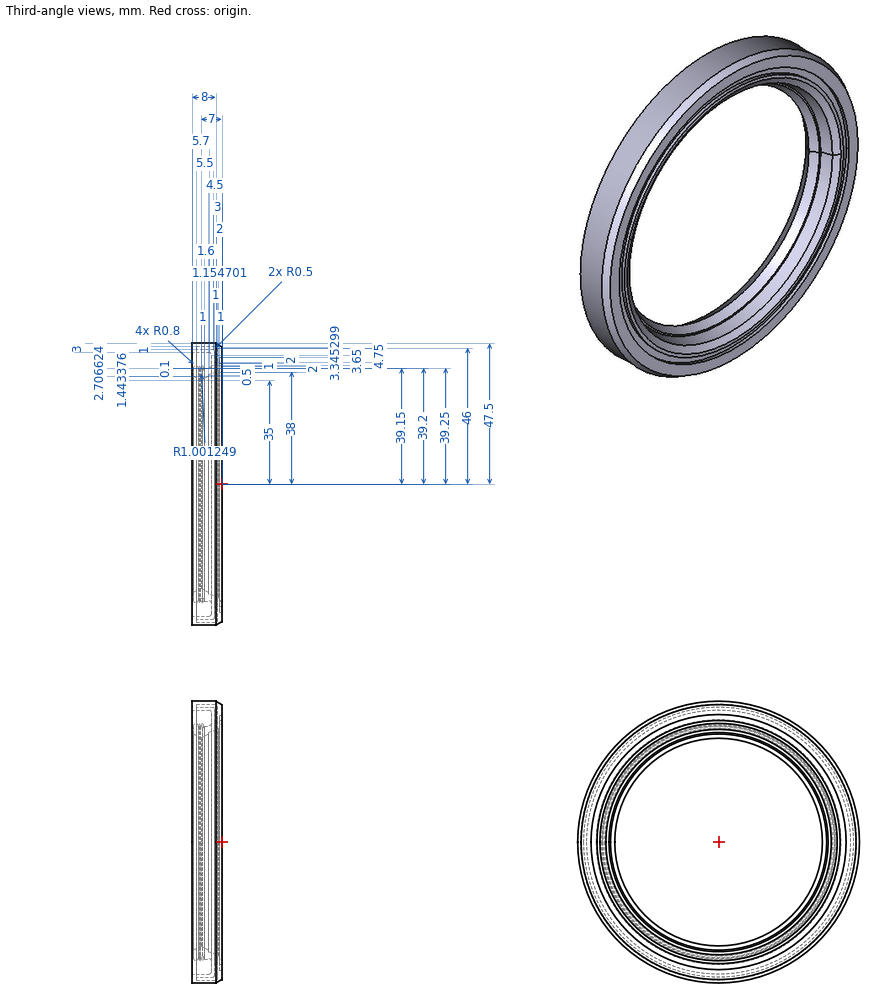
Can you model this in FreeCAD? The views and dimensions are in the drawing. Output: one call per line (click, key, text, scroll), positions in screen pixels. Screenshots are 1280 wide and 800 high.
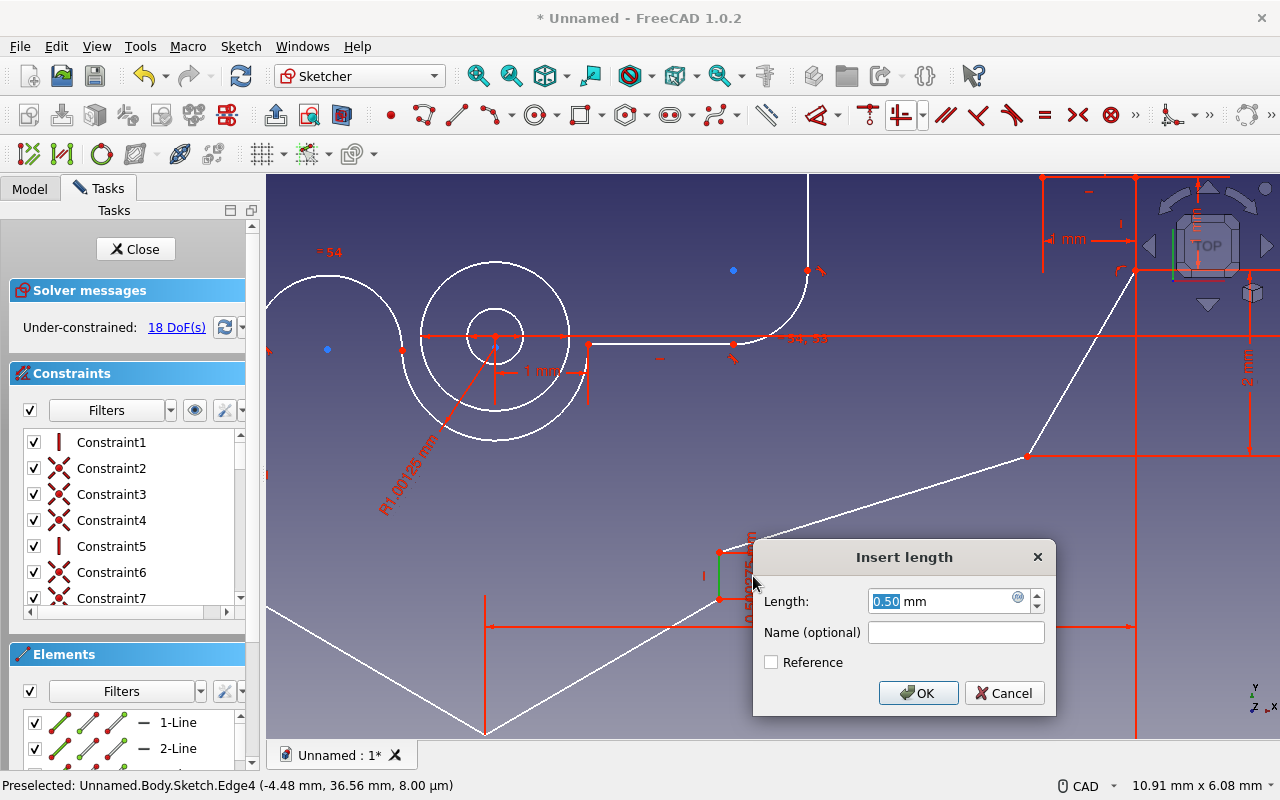
text(0.5)
key(Return)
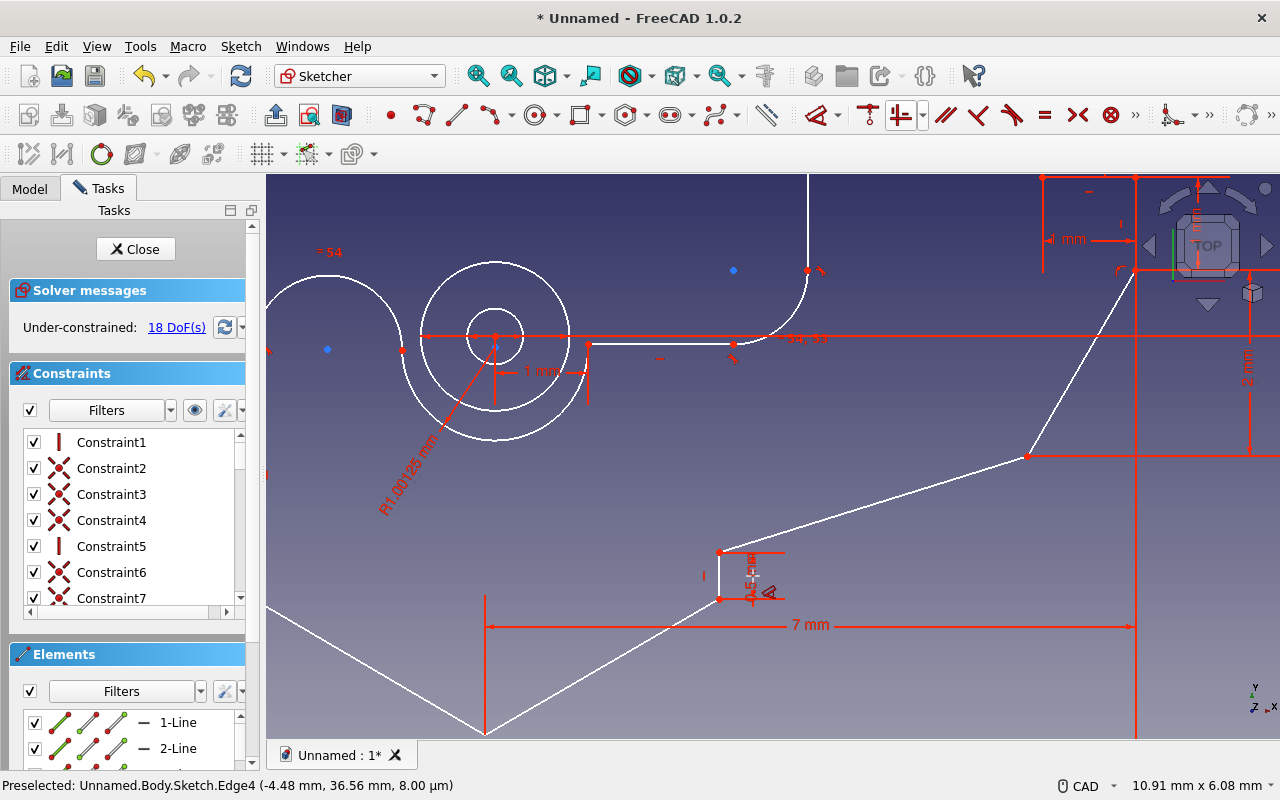
scroll(719, 588, down, 6)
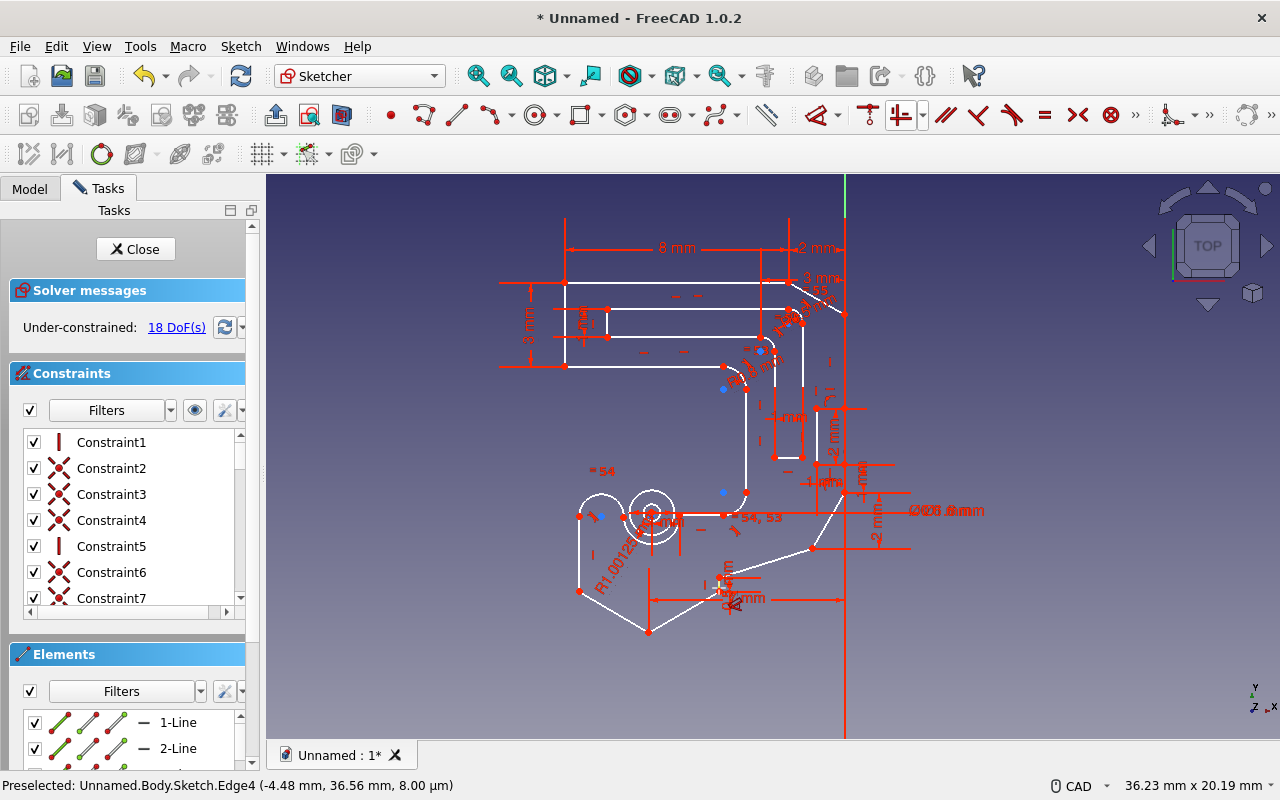
click(613, 367)
click(644, 401)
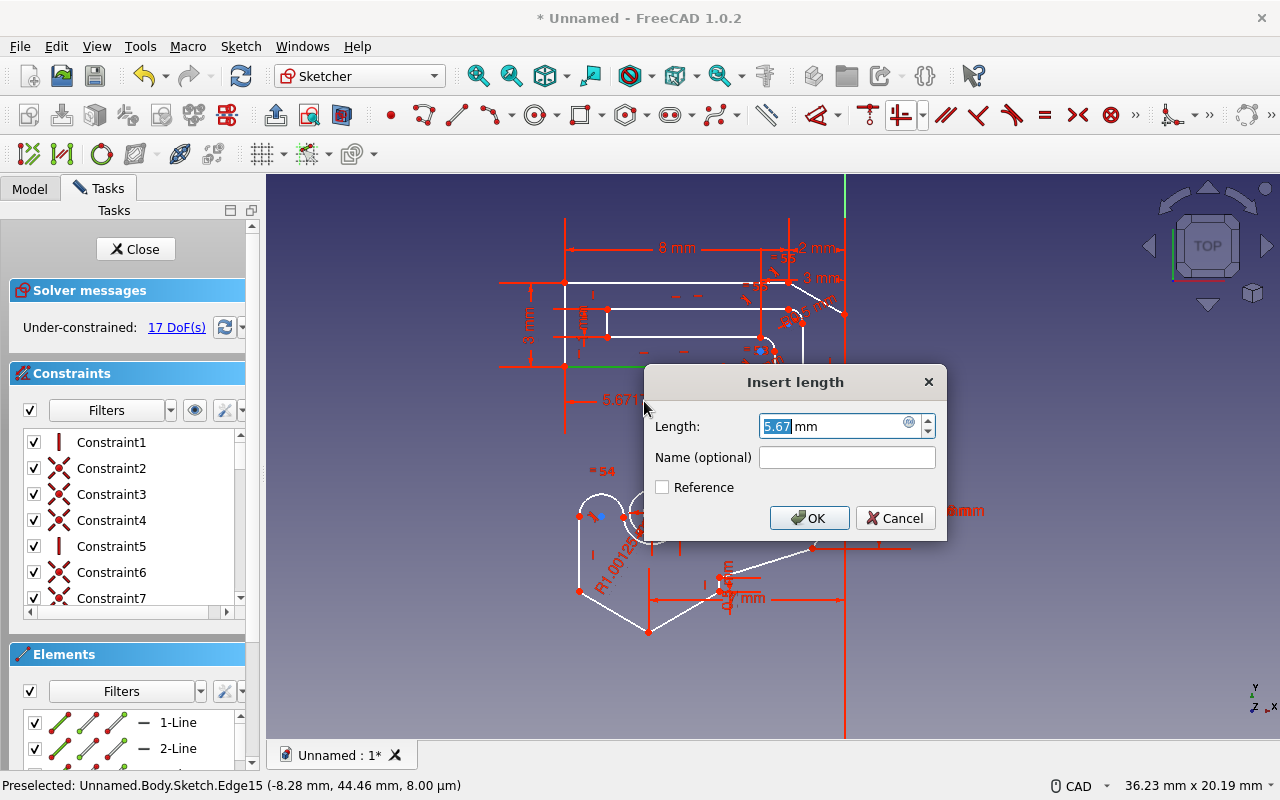
text(5.7)
key(Return)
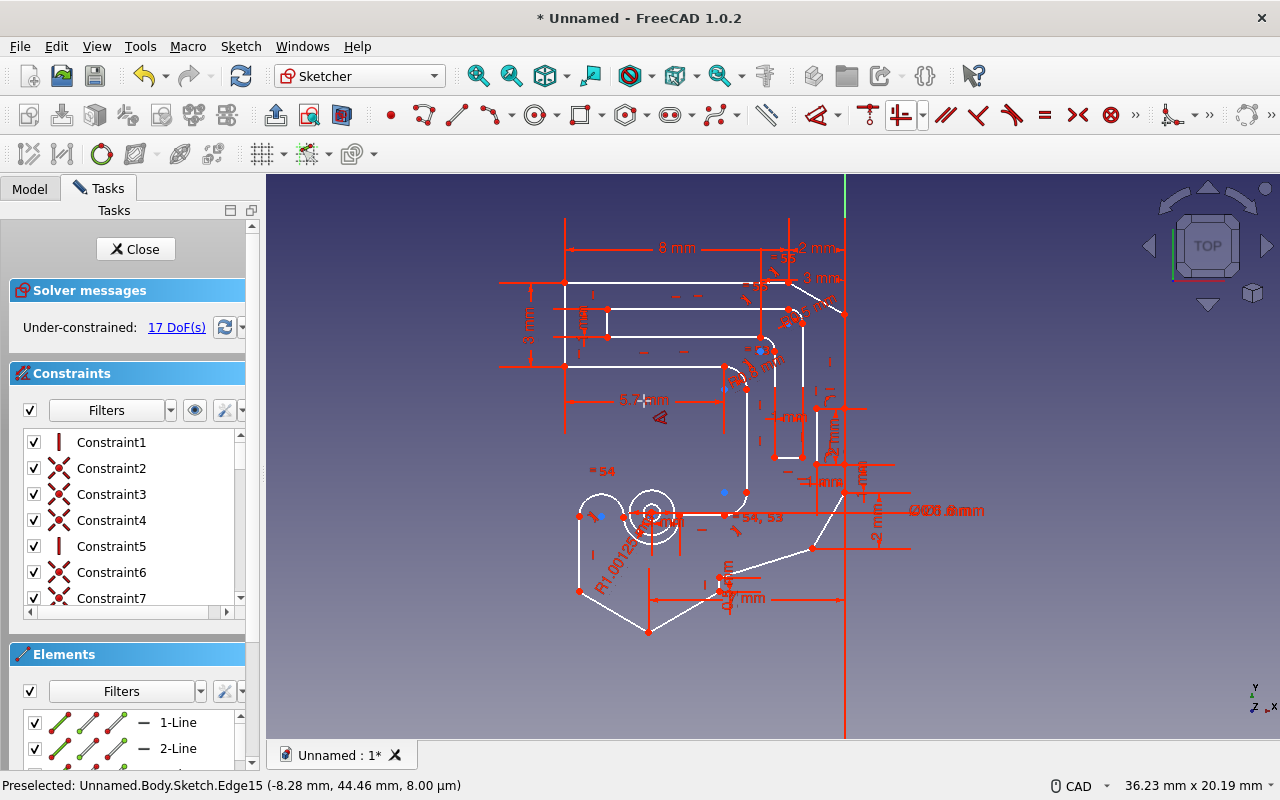
click(711, 515)
click(702, 549)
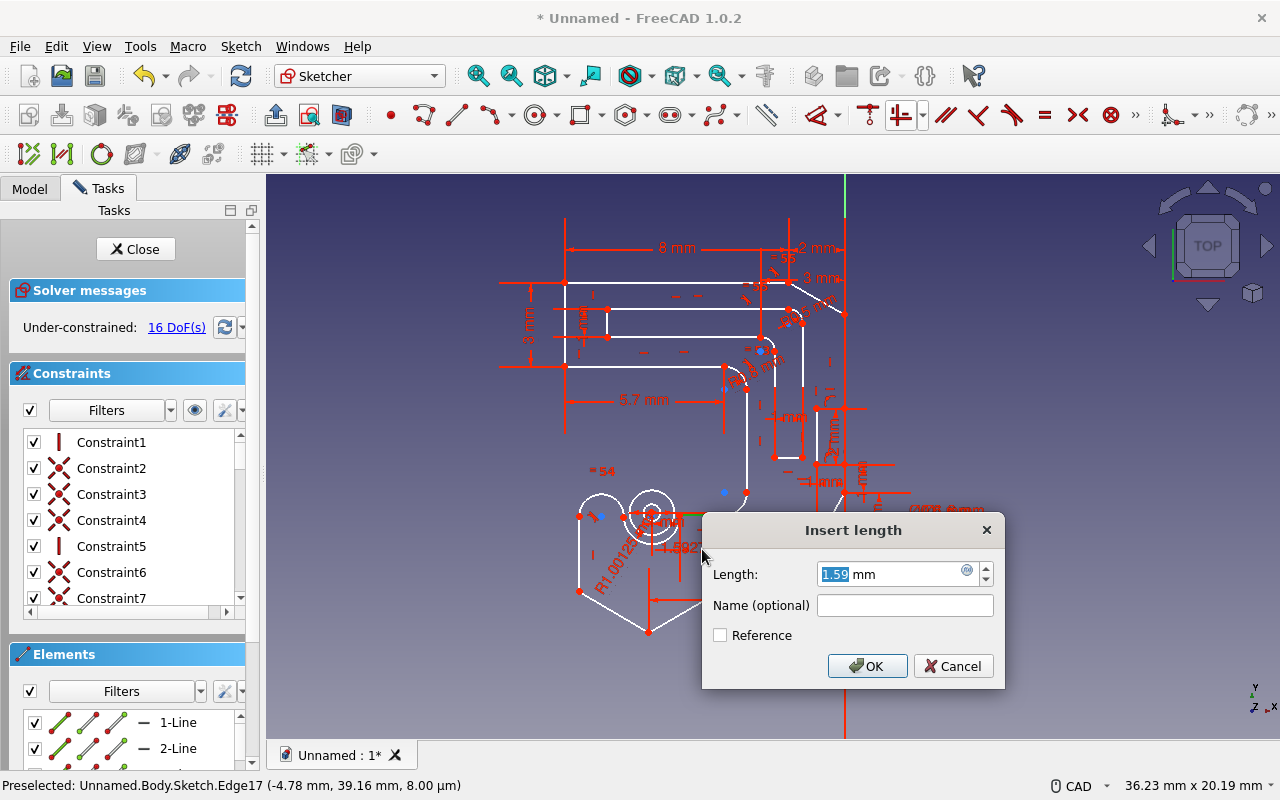
text(1.6)
key(Return)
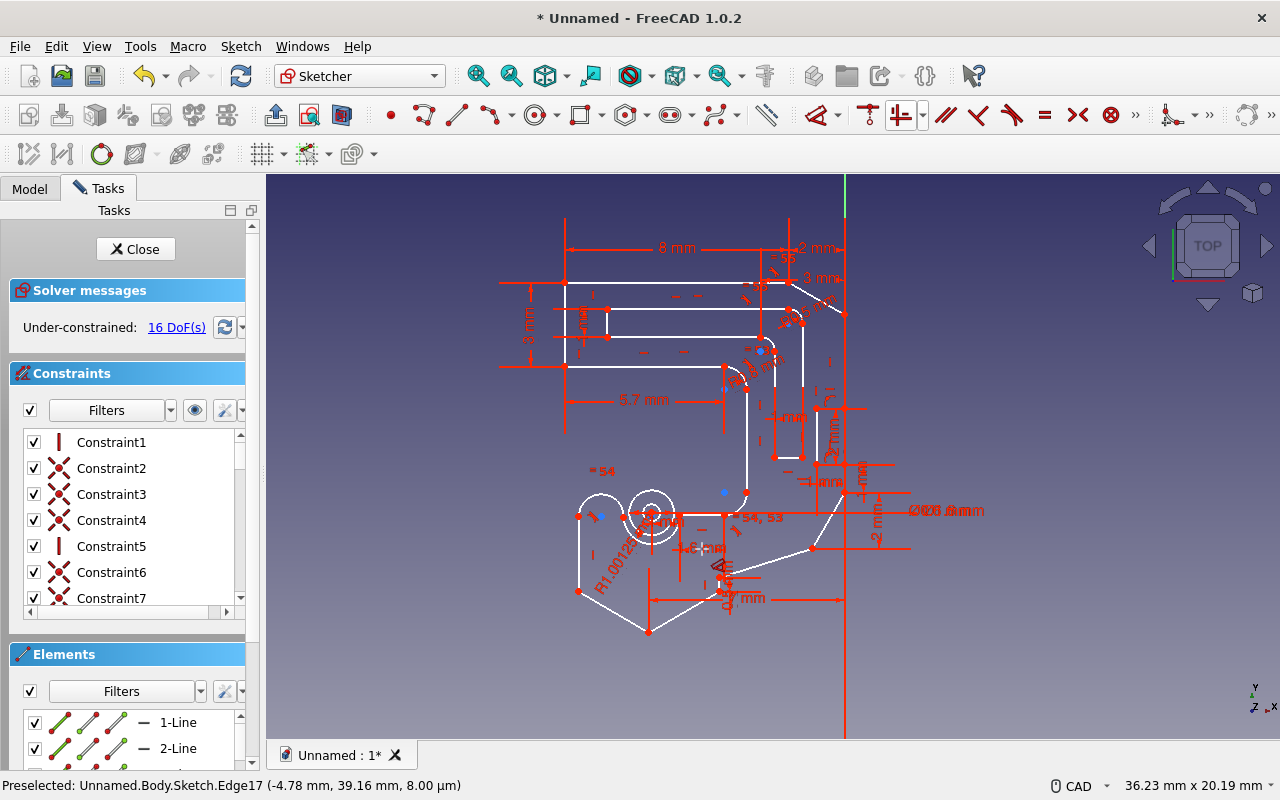
click(715, 337)
click(719, 395)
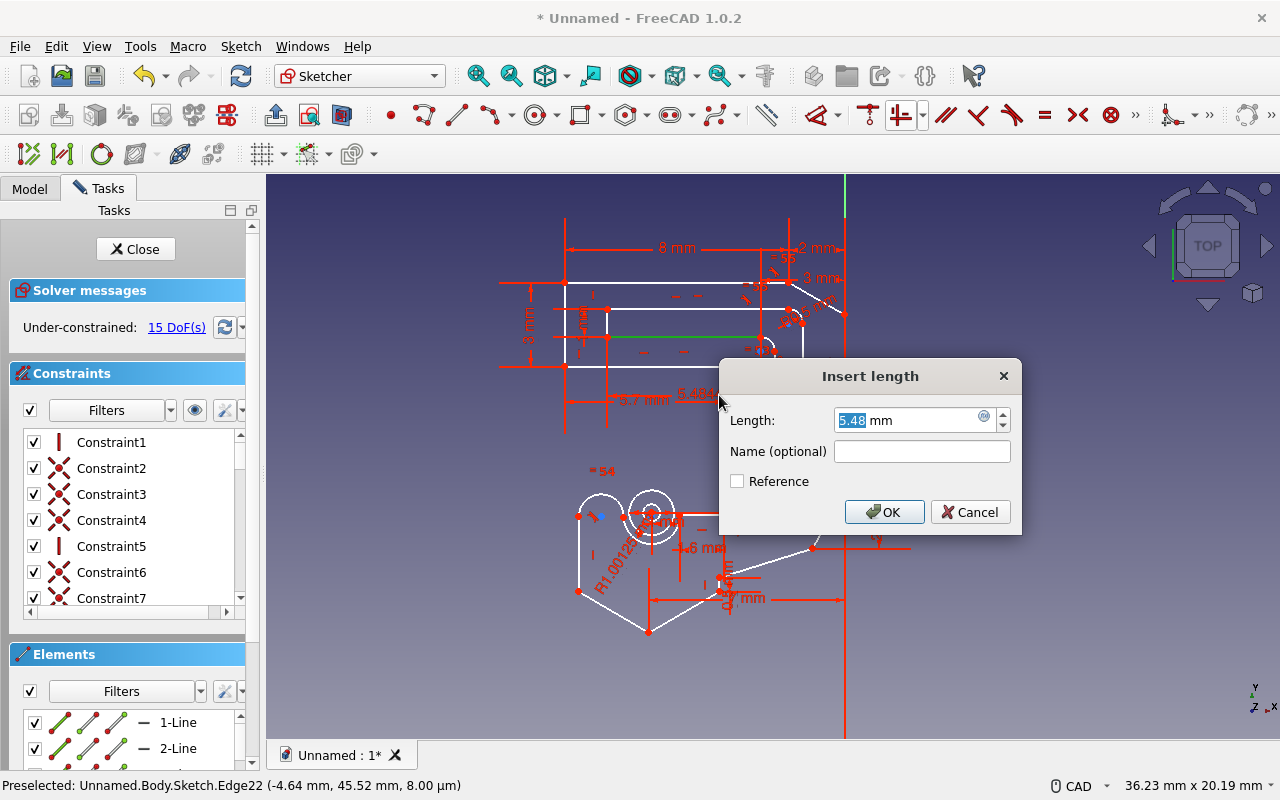
text(5.5)
key(Return)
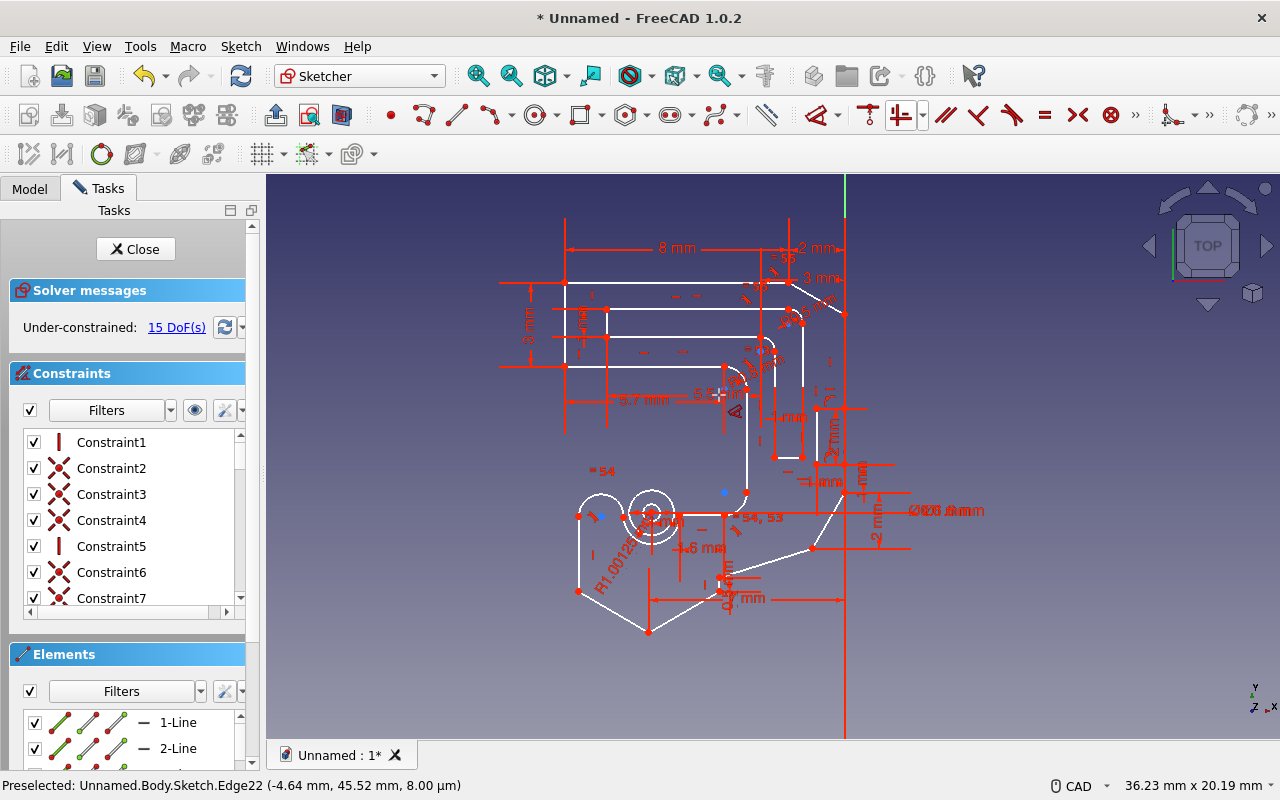
click(649, 633)
click(879, 672)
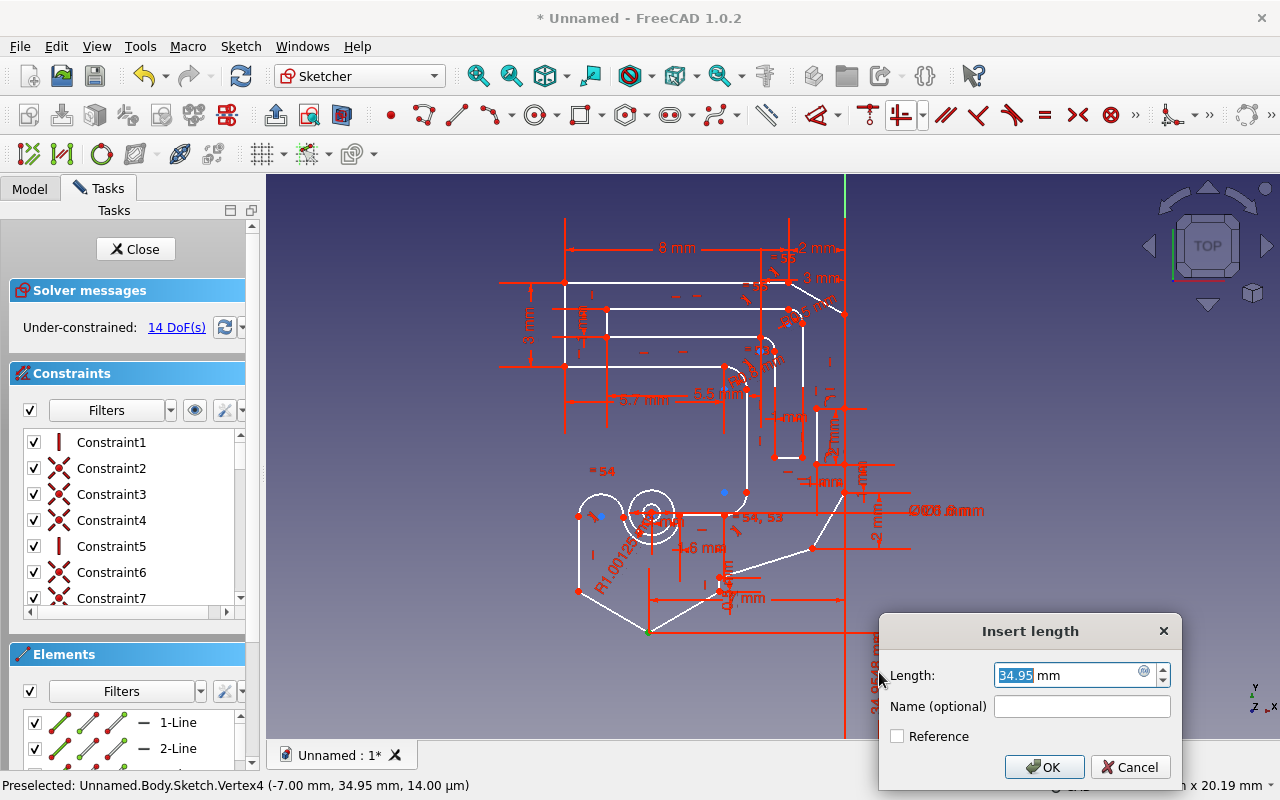
text(35)
key(Return)